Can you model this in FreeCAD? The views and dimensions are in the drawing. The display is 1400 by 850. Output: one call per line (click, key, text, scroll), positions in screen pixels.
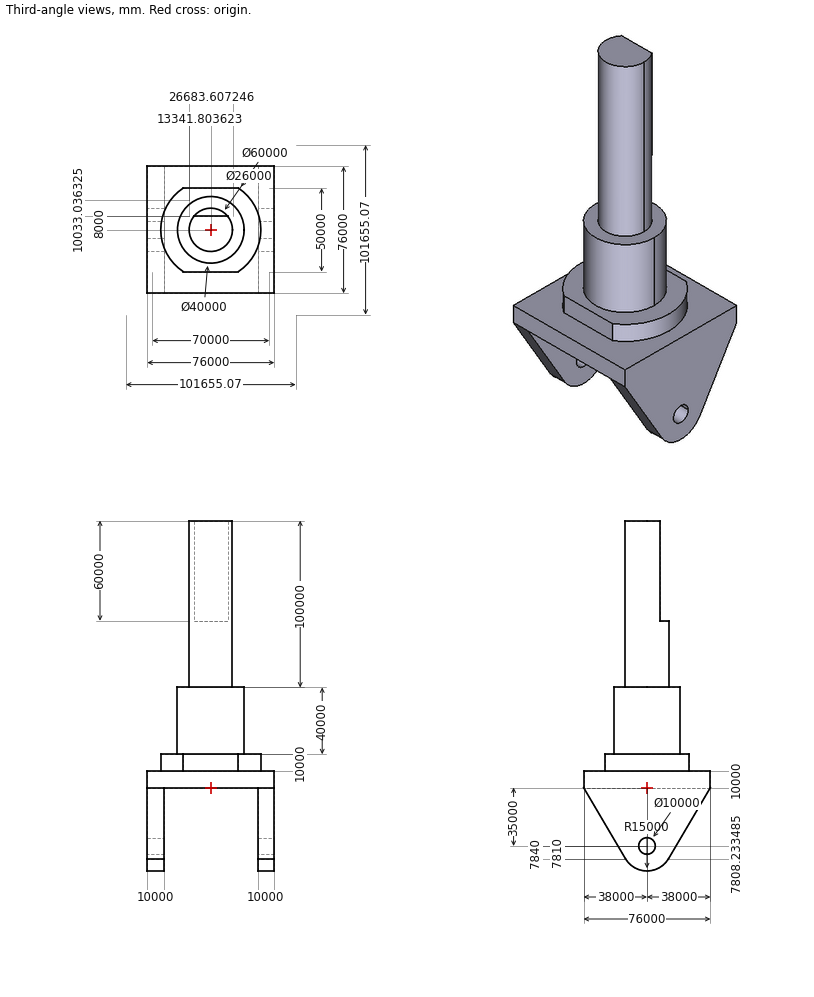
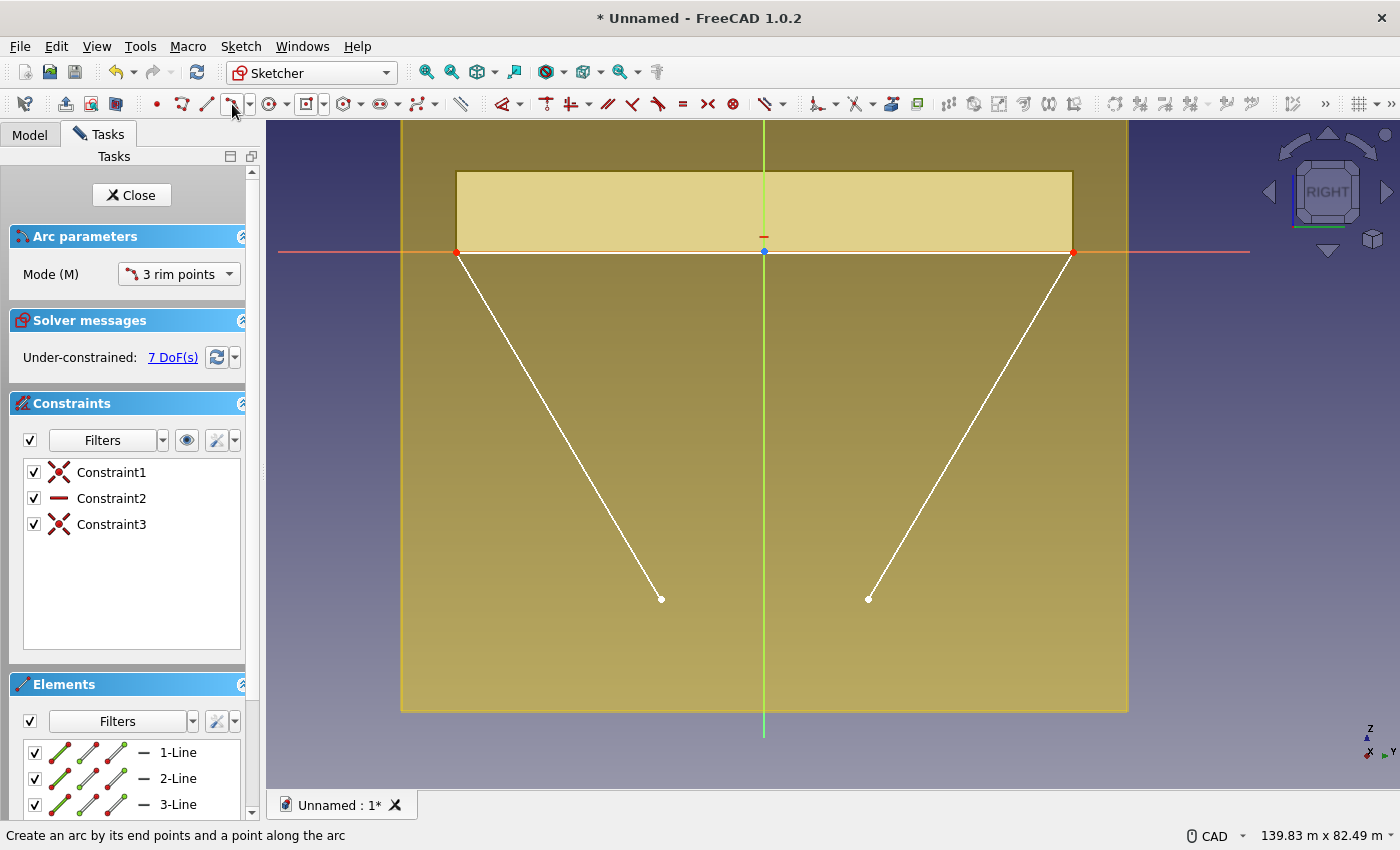
click(868, 600)
click(661, 600)
click(740, 655)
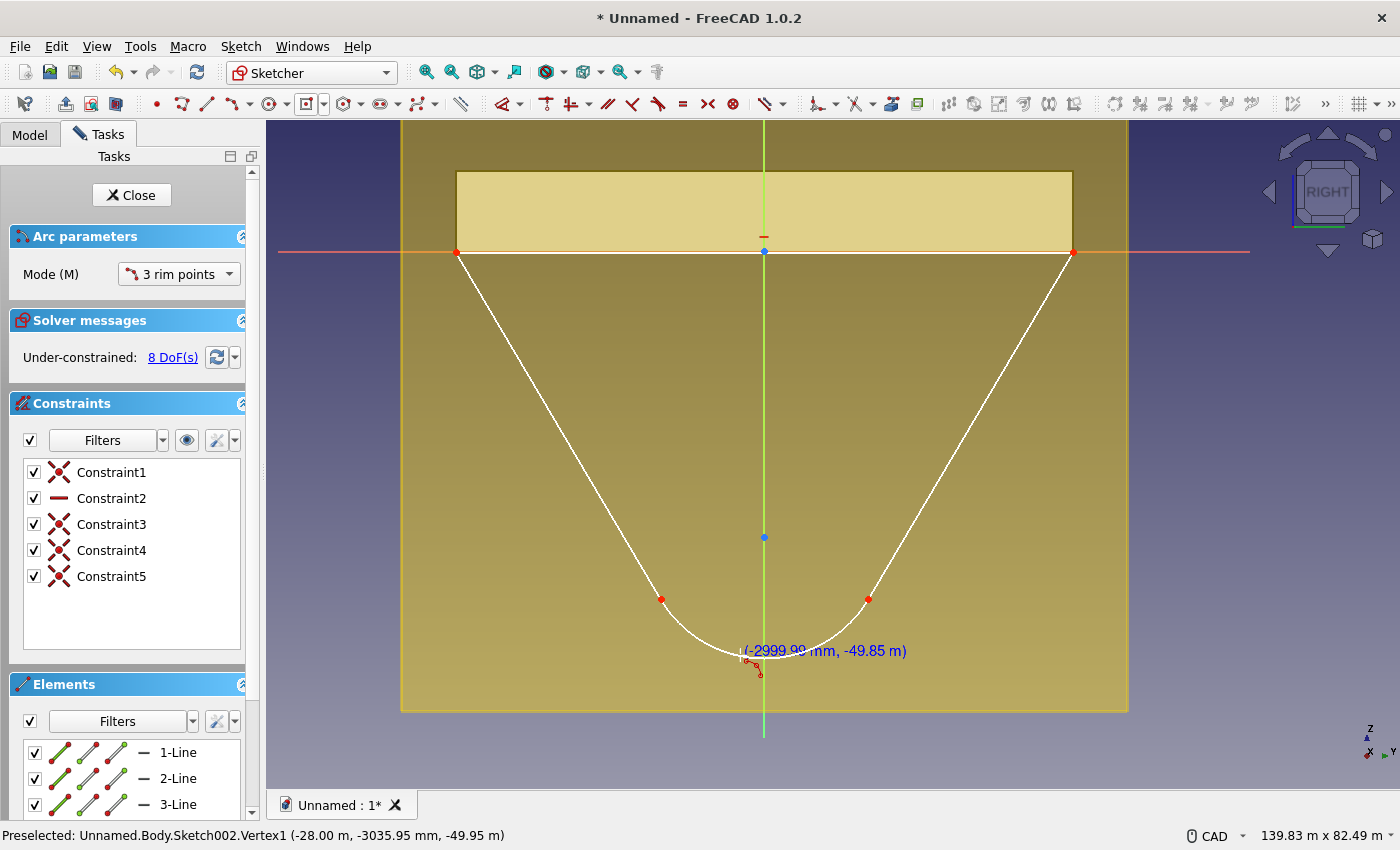
click(268, 104)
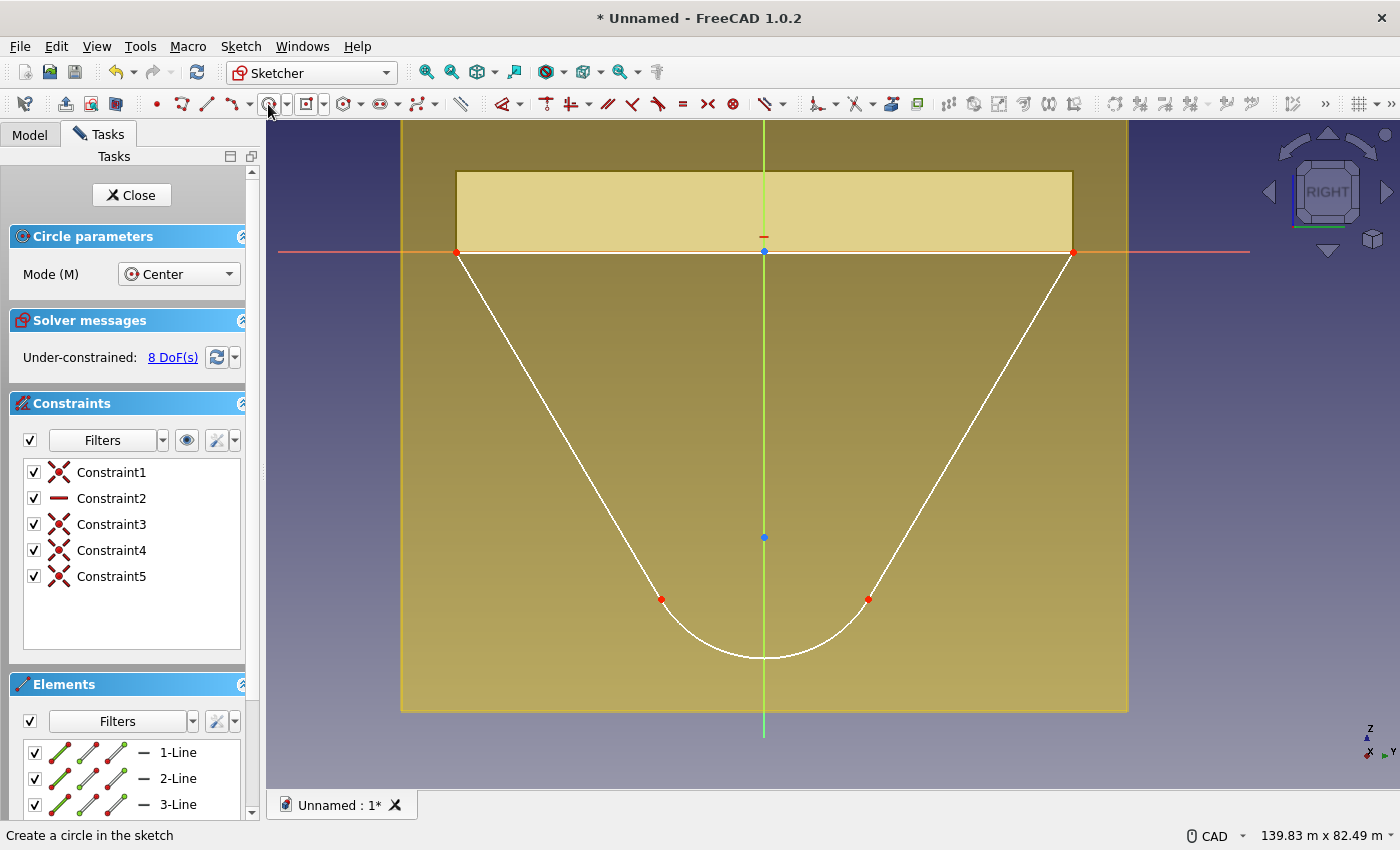
click(764, 536)
click(793, 507)
key(Escape)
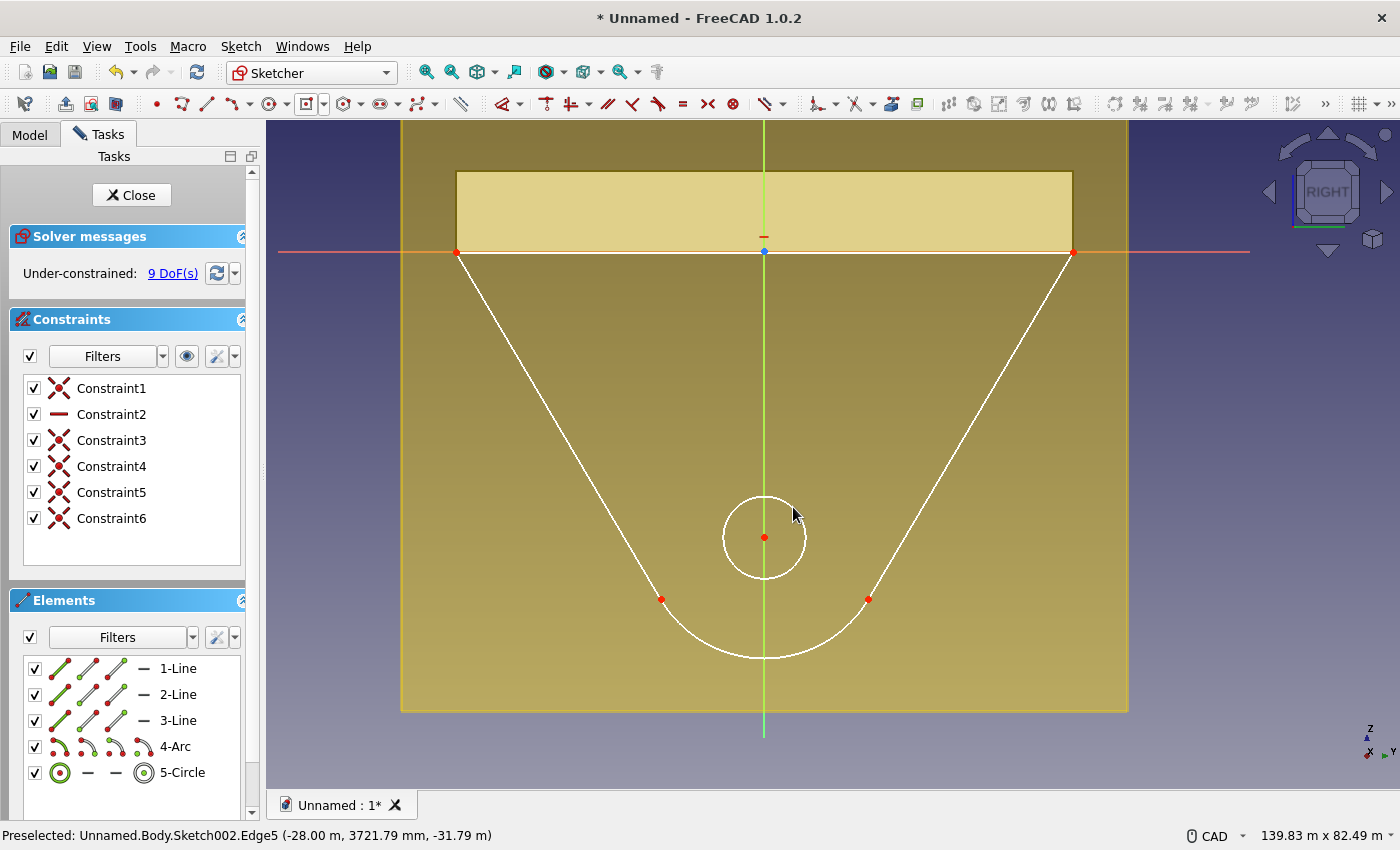
click(764, 538)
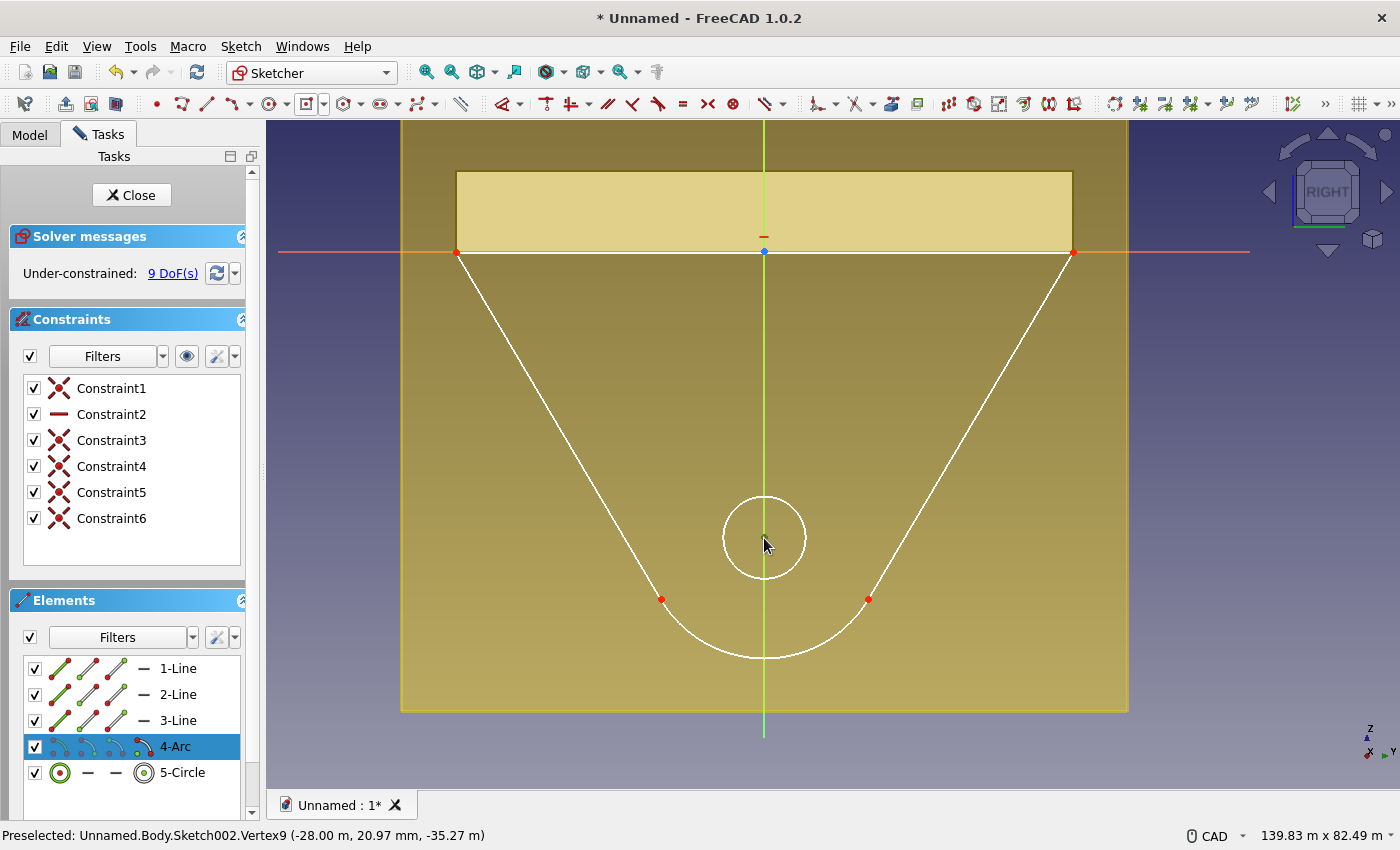
click(764, 717)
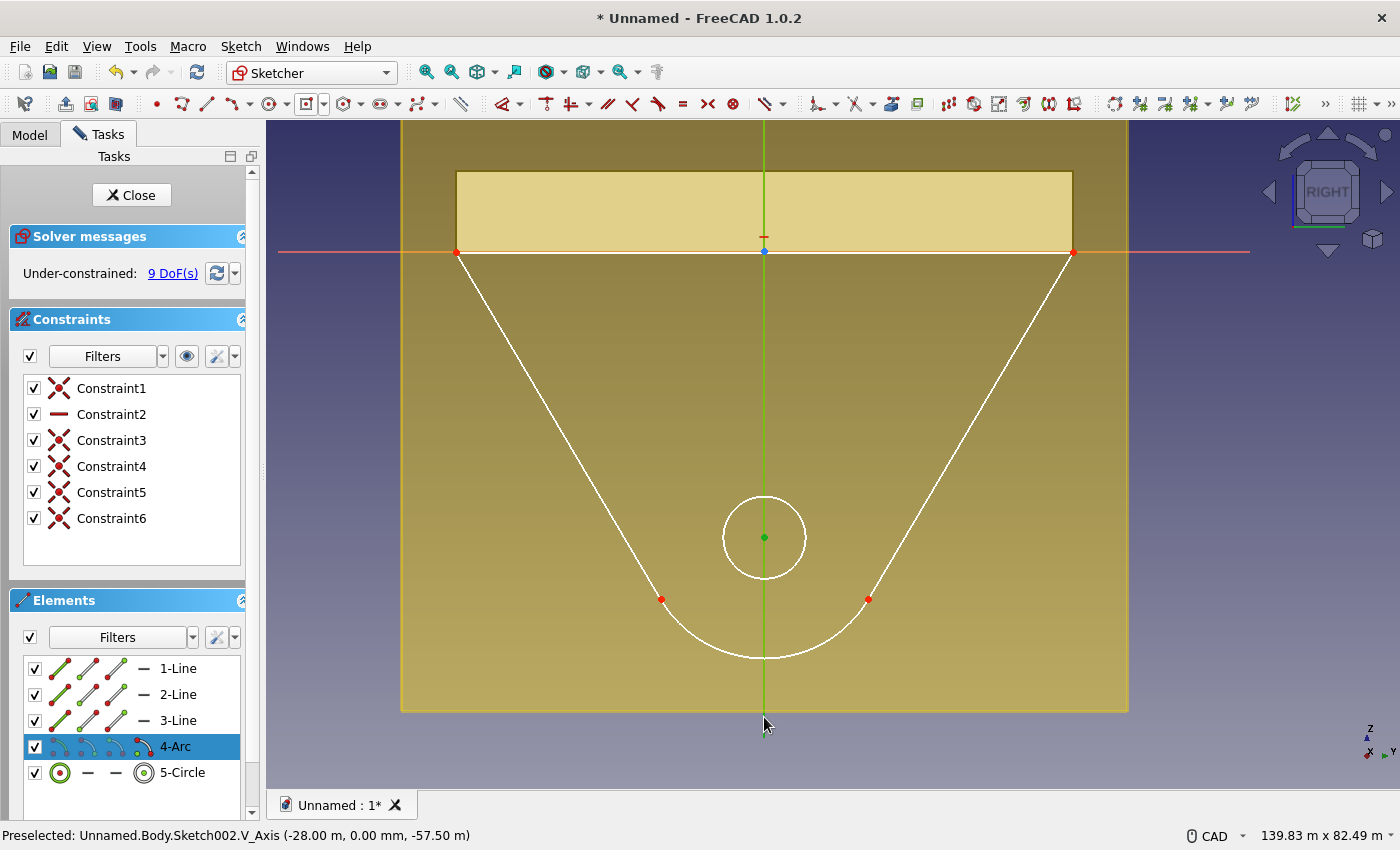
key(c)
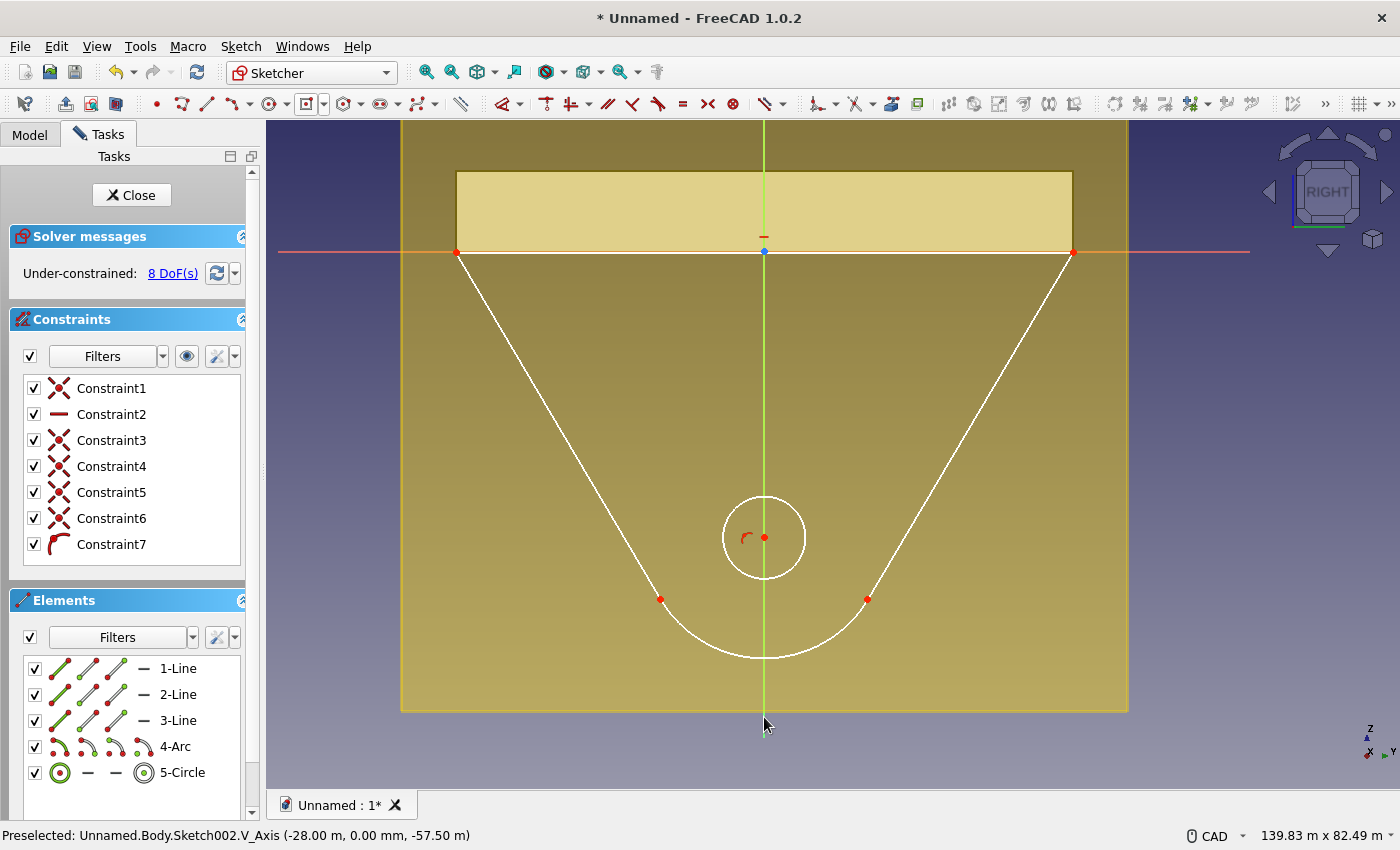
click(502, 104)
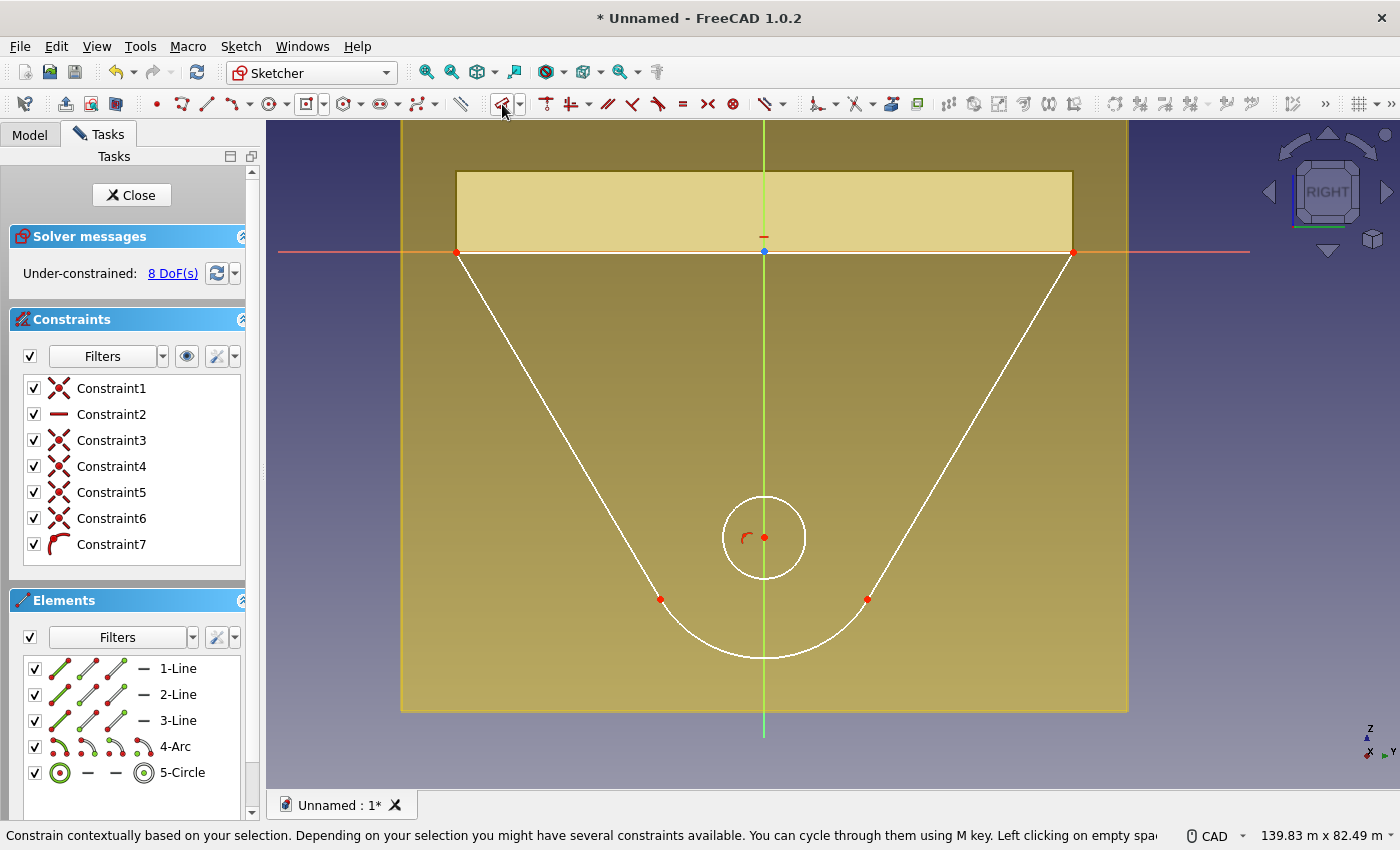
click(716, 648)
click(703, 677)